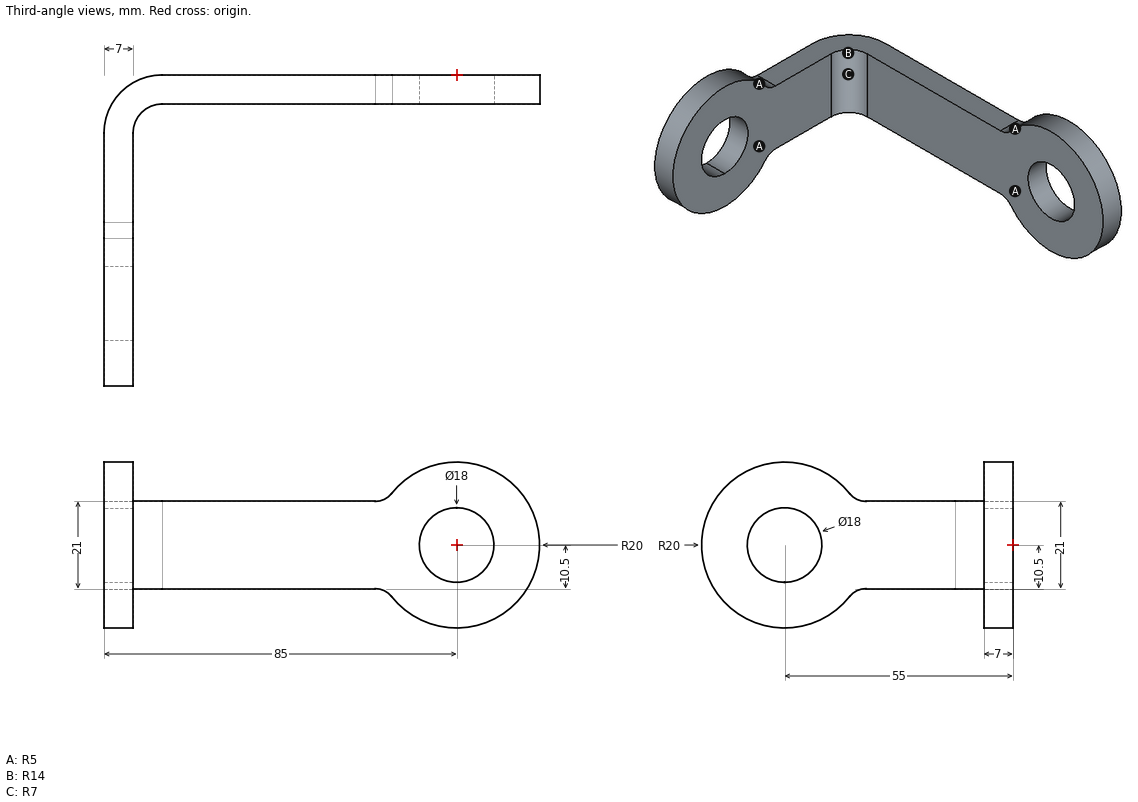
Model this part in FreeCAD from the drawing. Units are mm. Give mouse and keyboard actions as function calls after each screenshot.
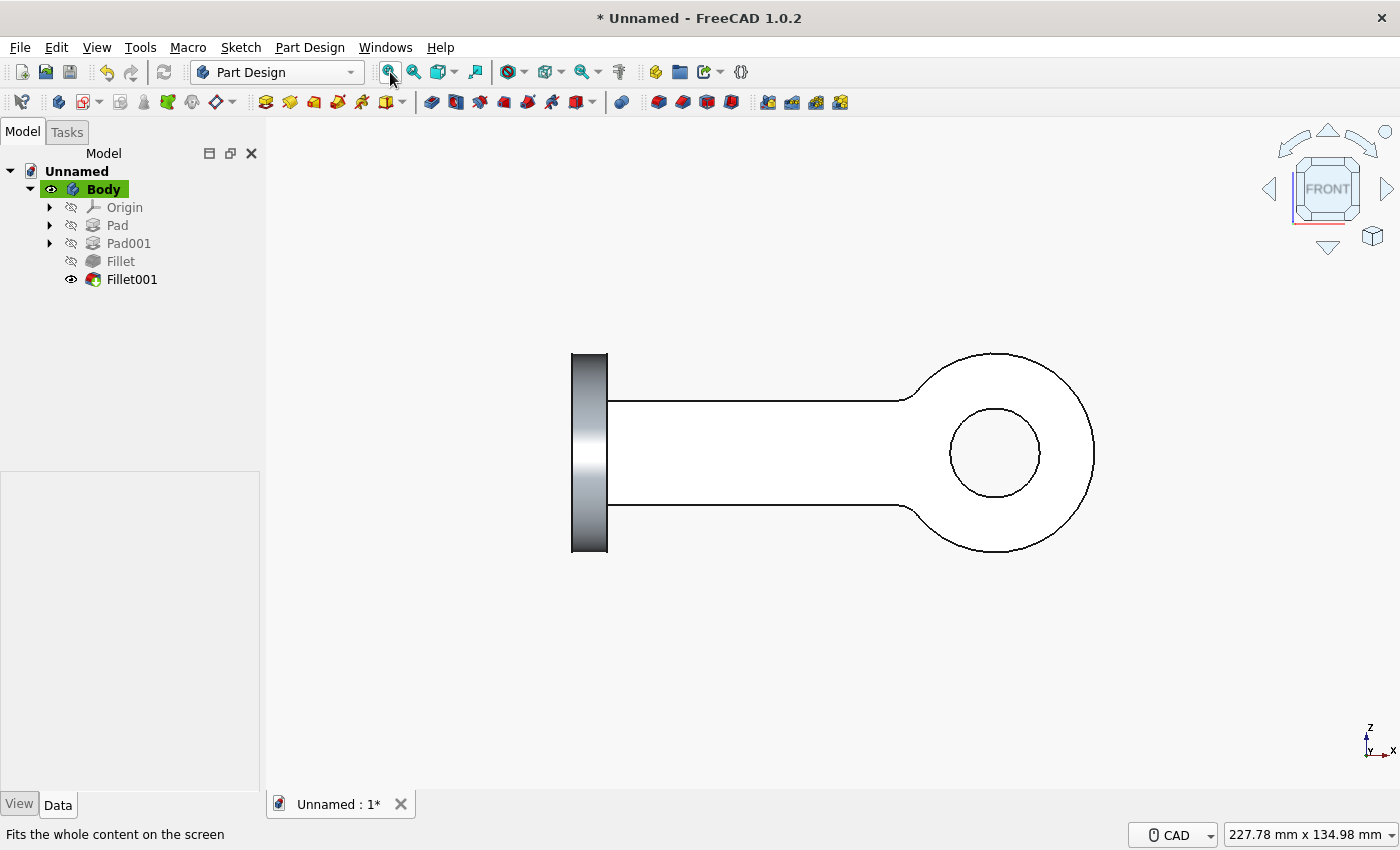
key(3)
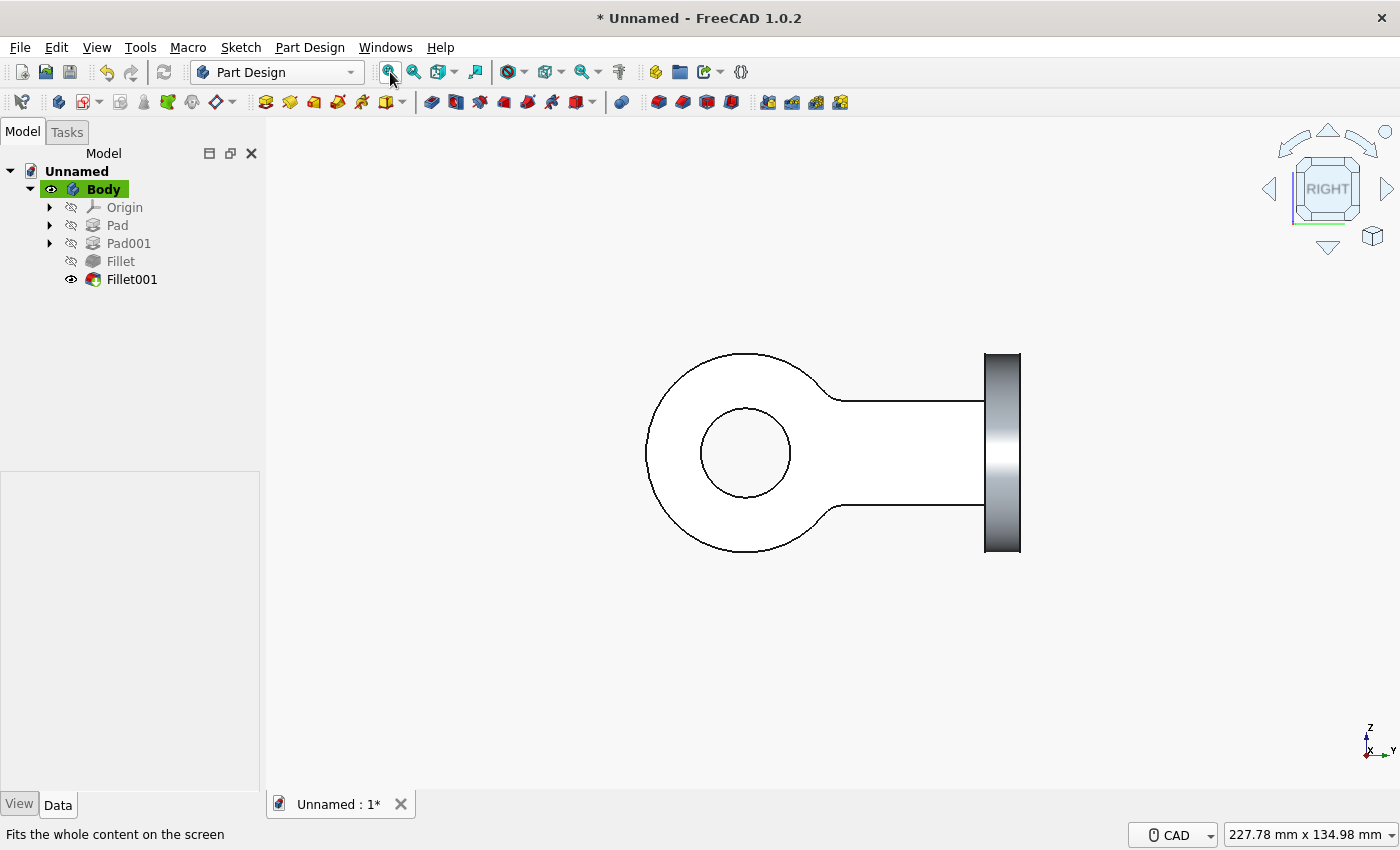
click(390, 72)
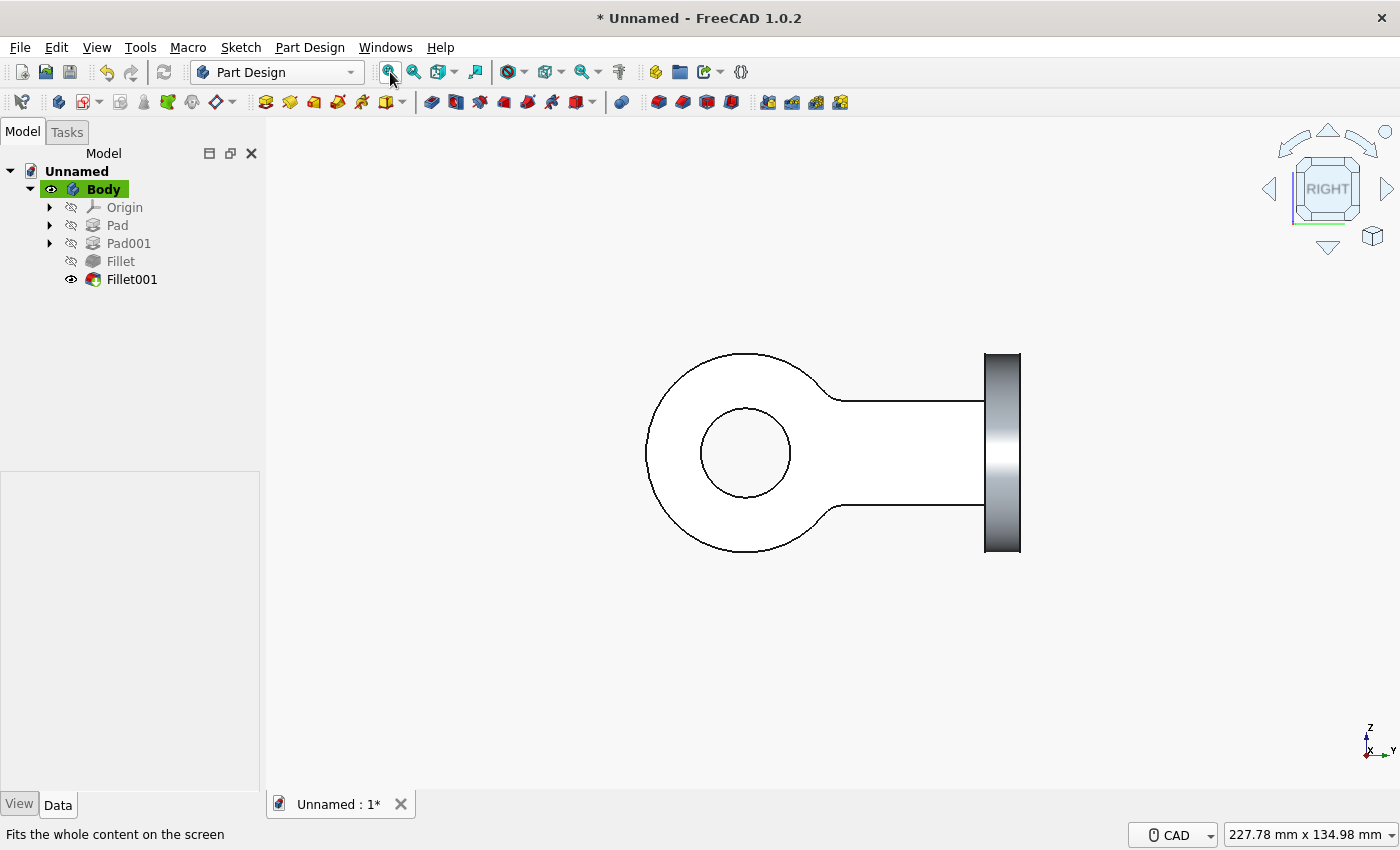
key(5)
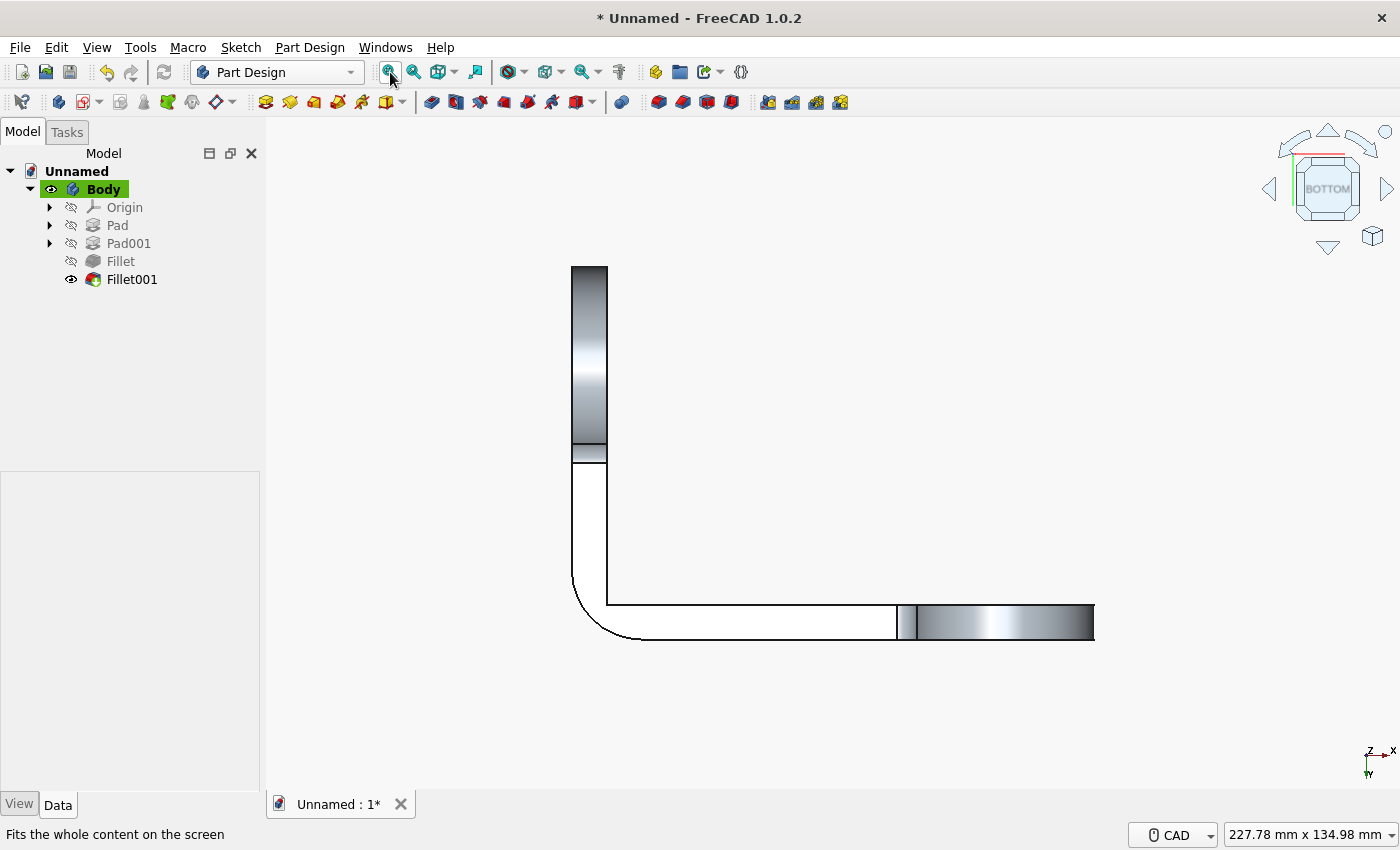
key(4)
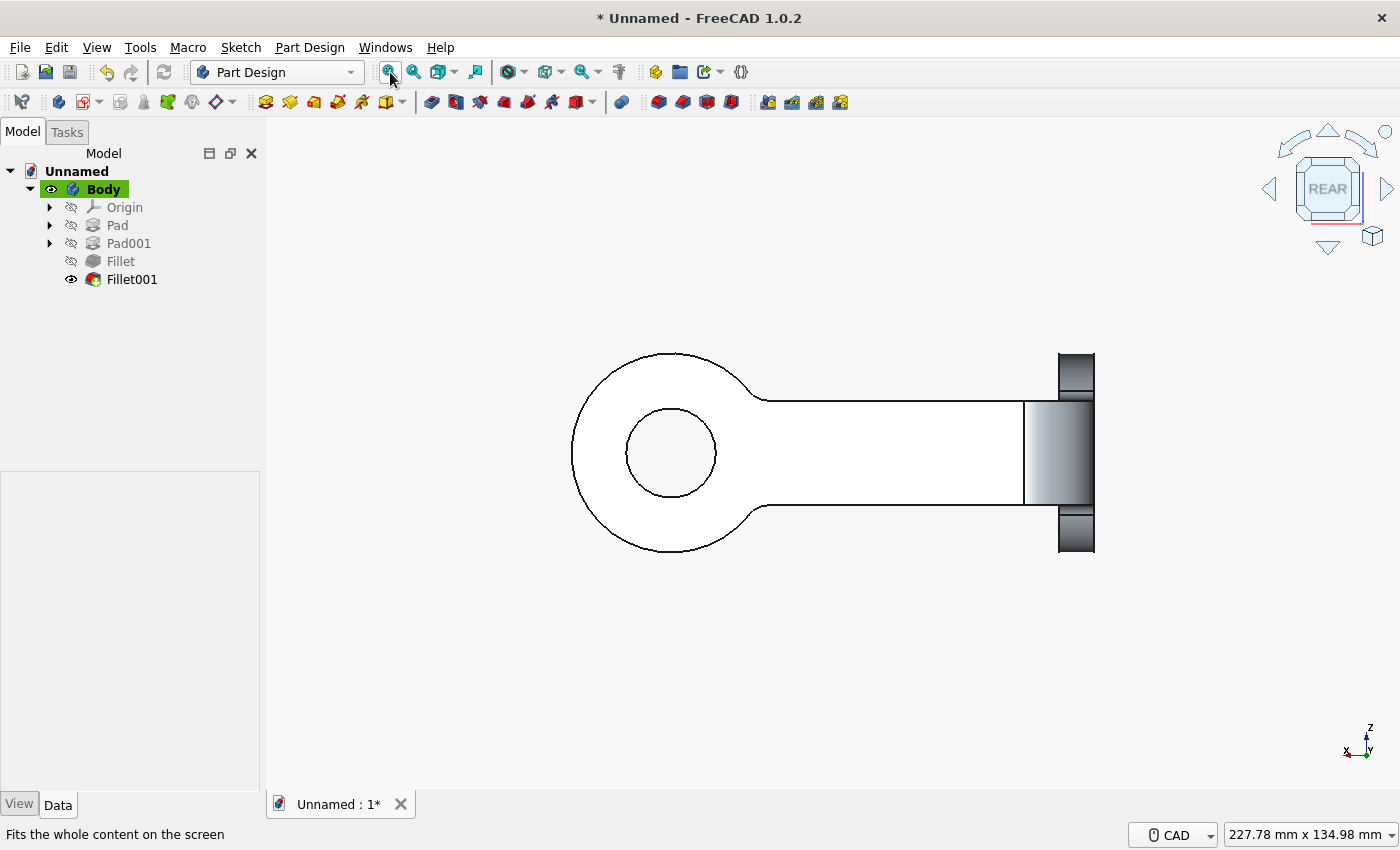
key(6)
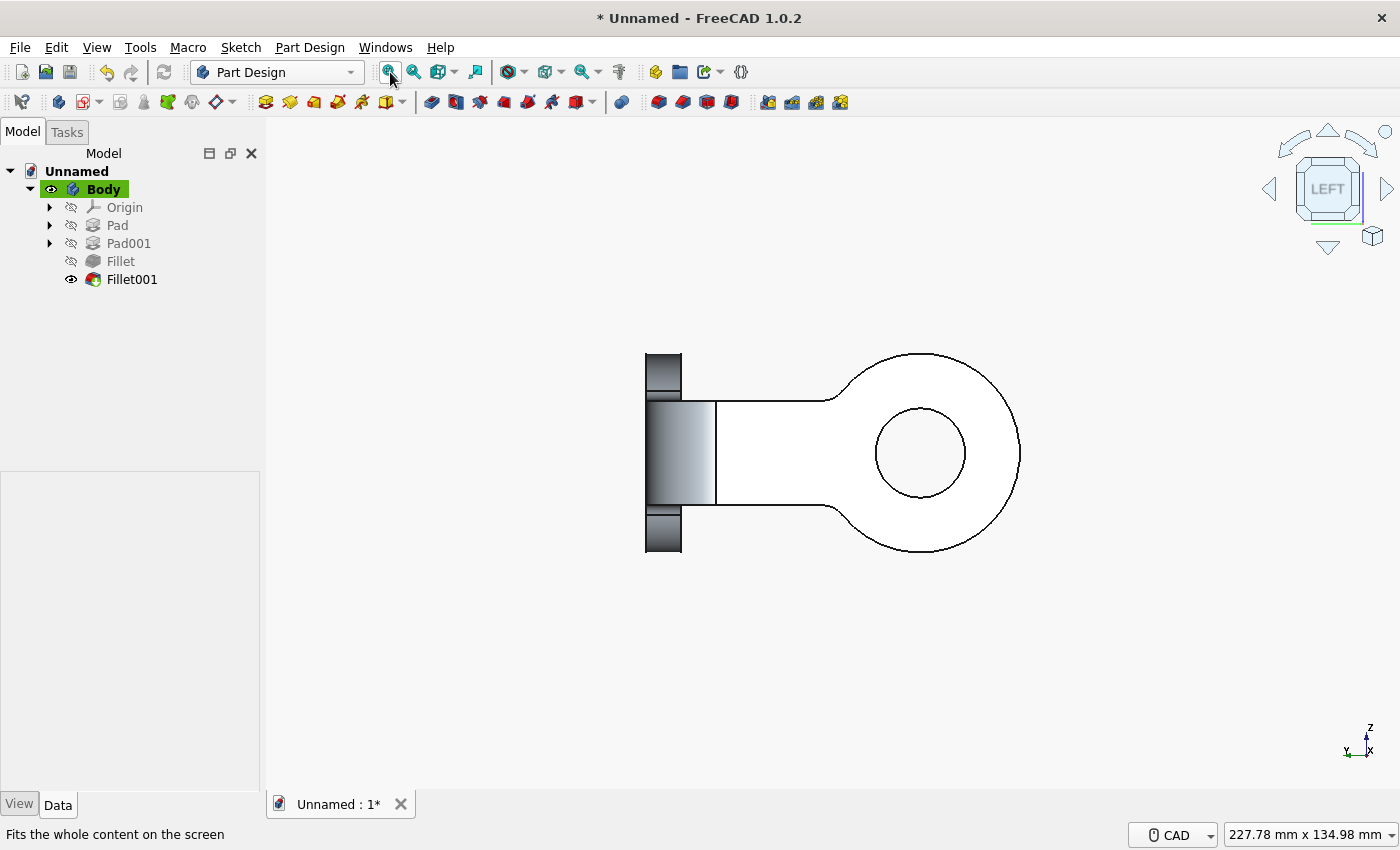
click(390, 72)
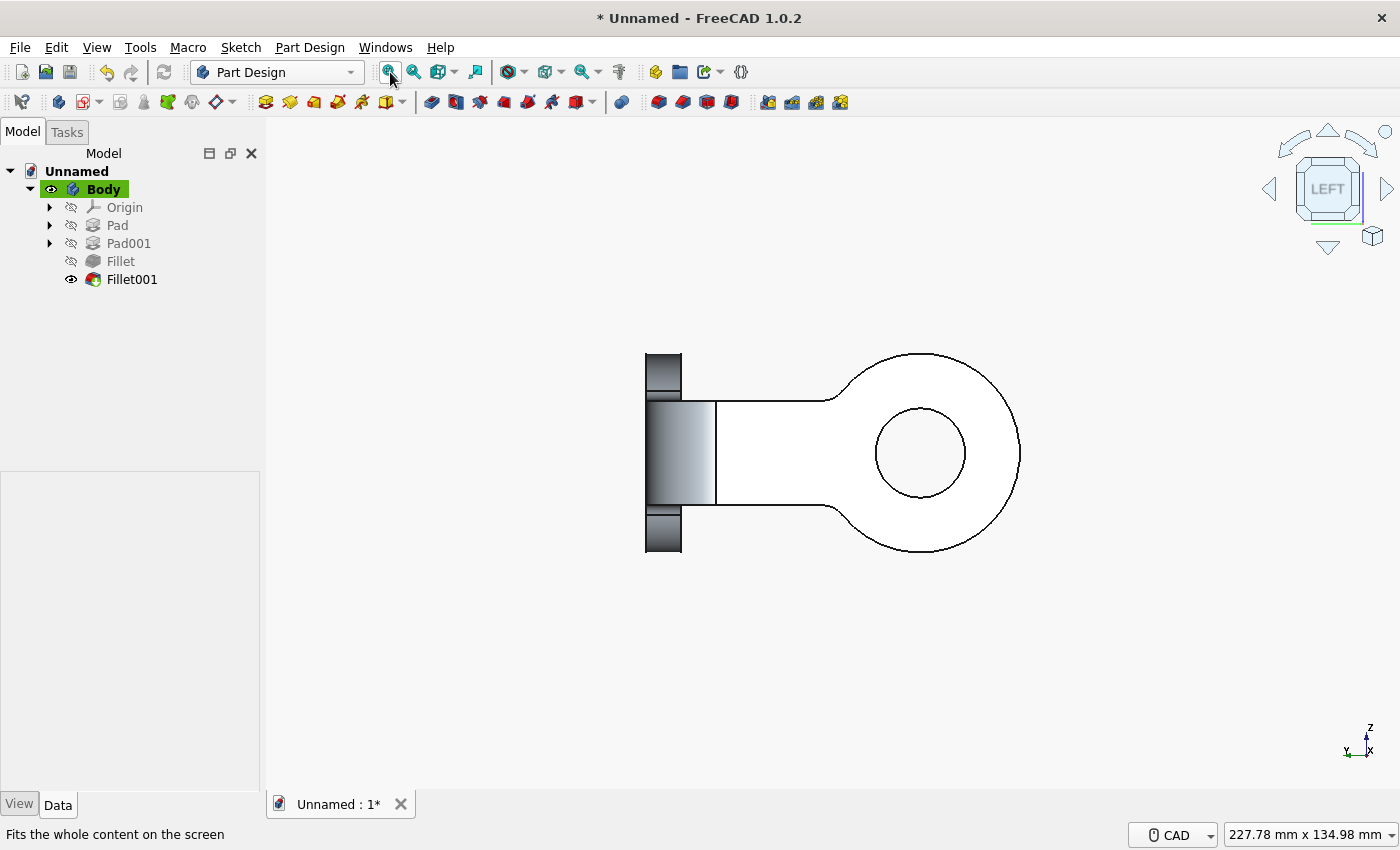
key(v)
key(3)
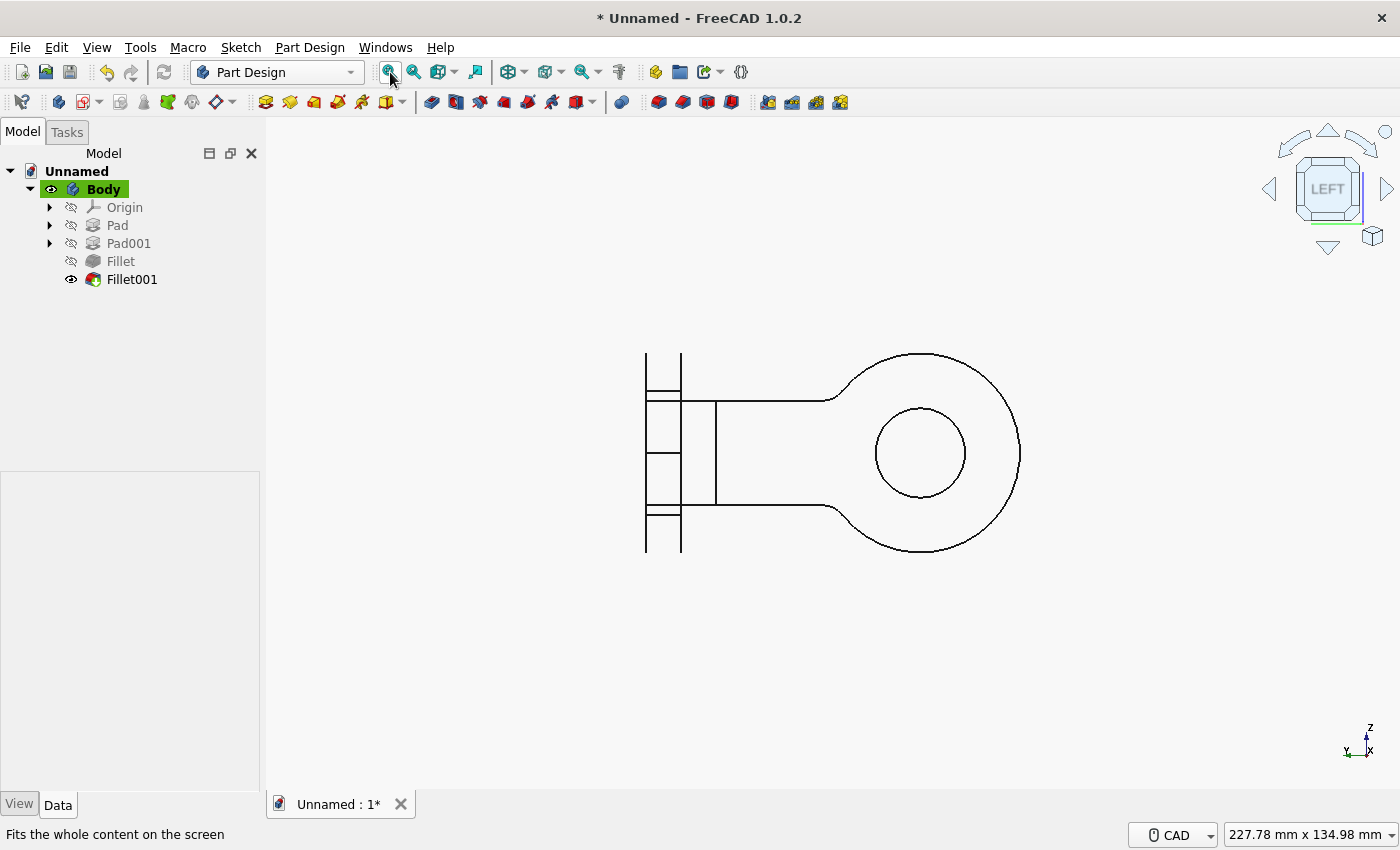
key(0)